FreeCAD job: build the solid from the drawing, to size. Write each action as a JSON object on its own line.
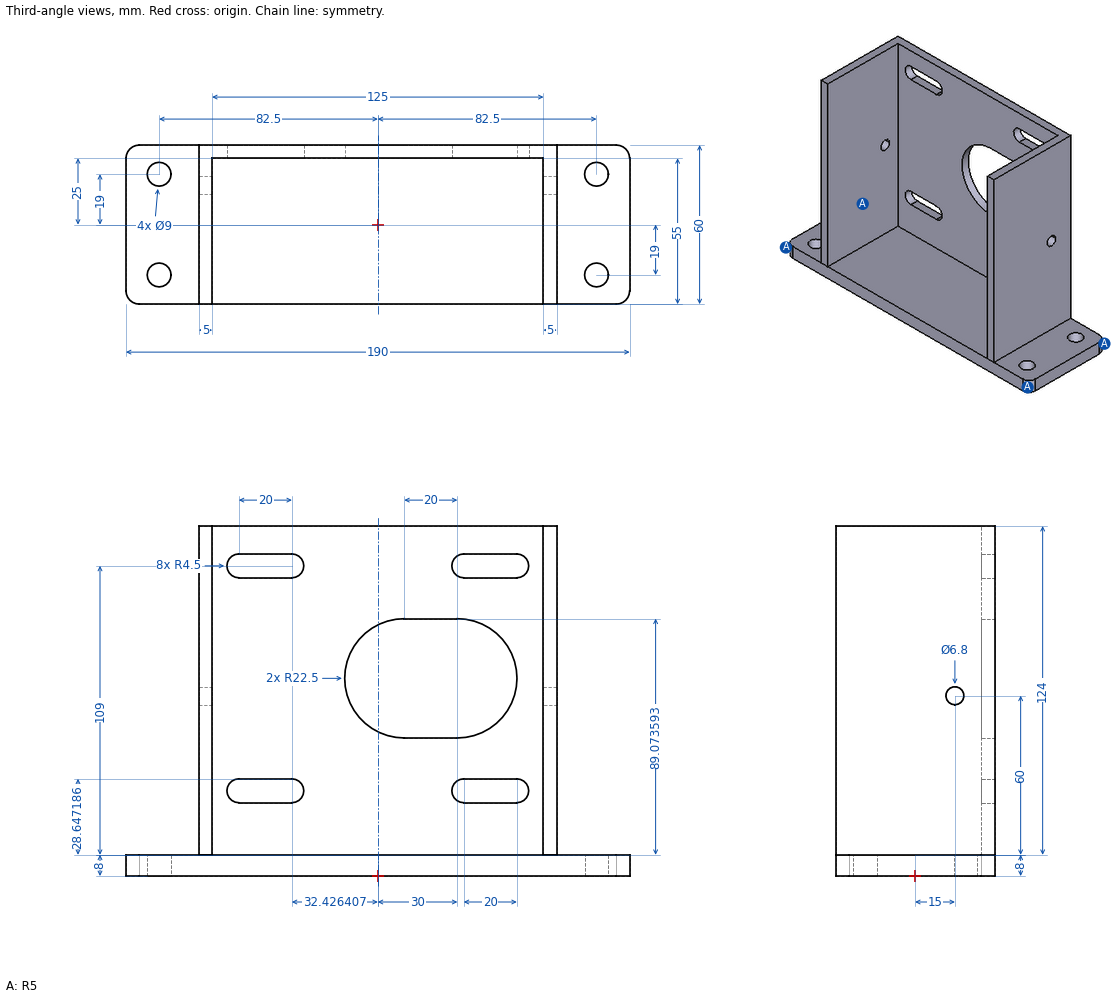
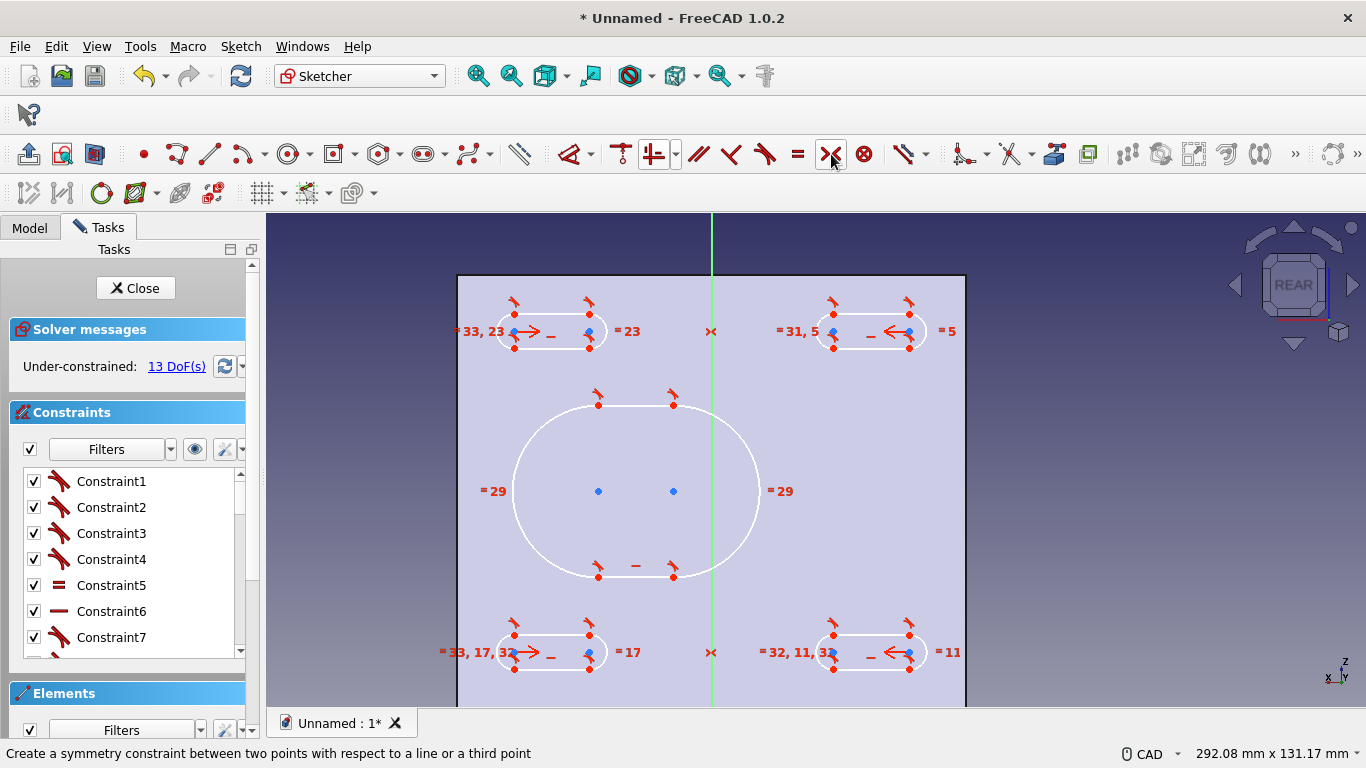
{"action": "left_click", "coordinate": [568, 154]}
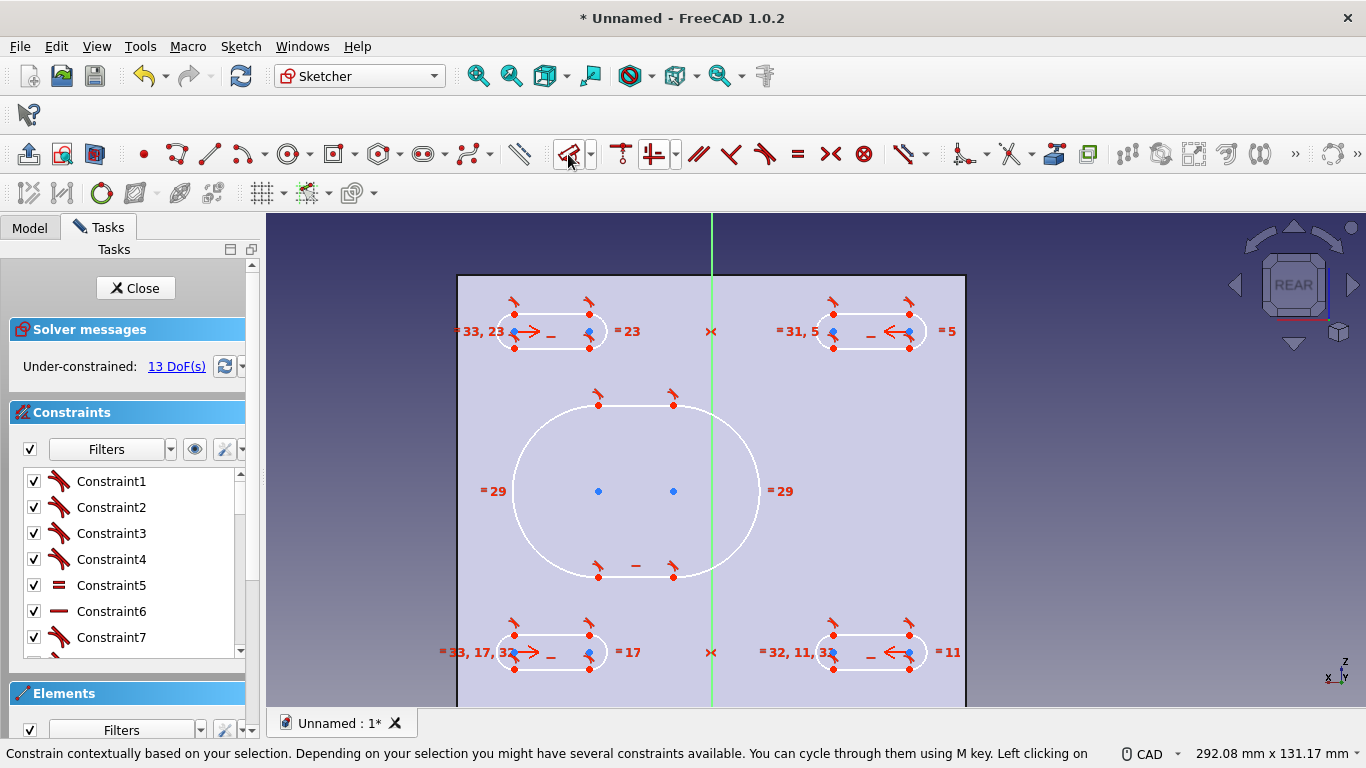
{"action": "scroll", "coordinate": [820, 321], "scroll_direction": "up", "scroll_amount": 5}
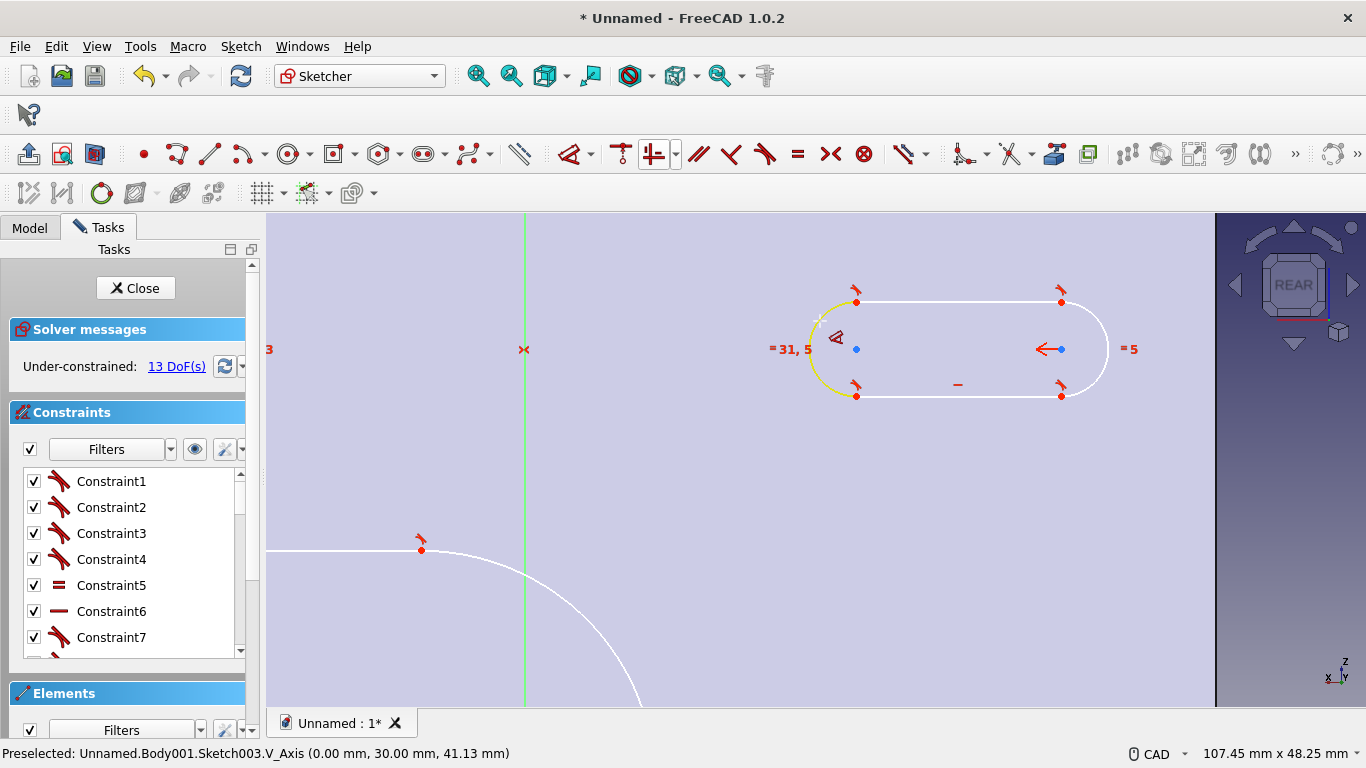
{"action": "left_click", "coordinate": [818, 322]}
{"action": "left_click", "coordinate": [792, 303]}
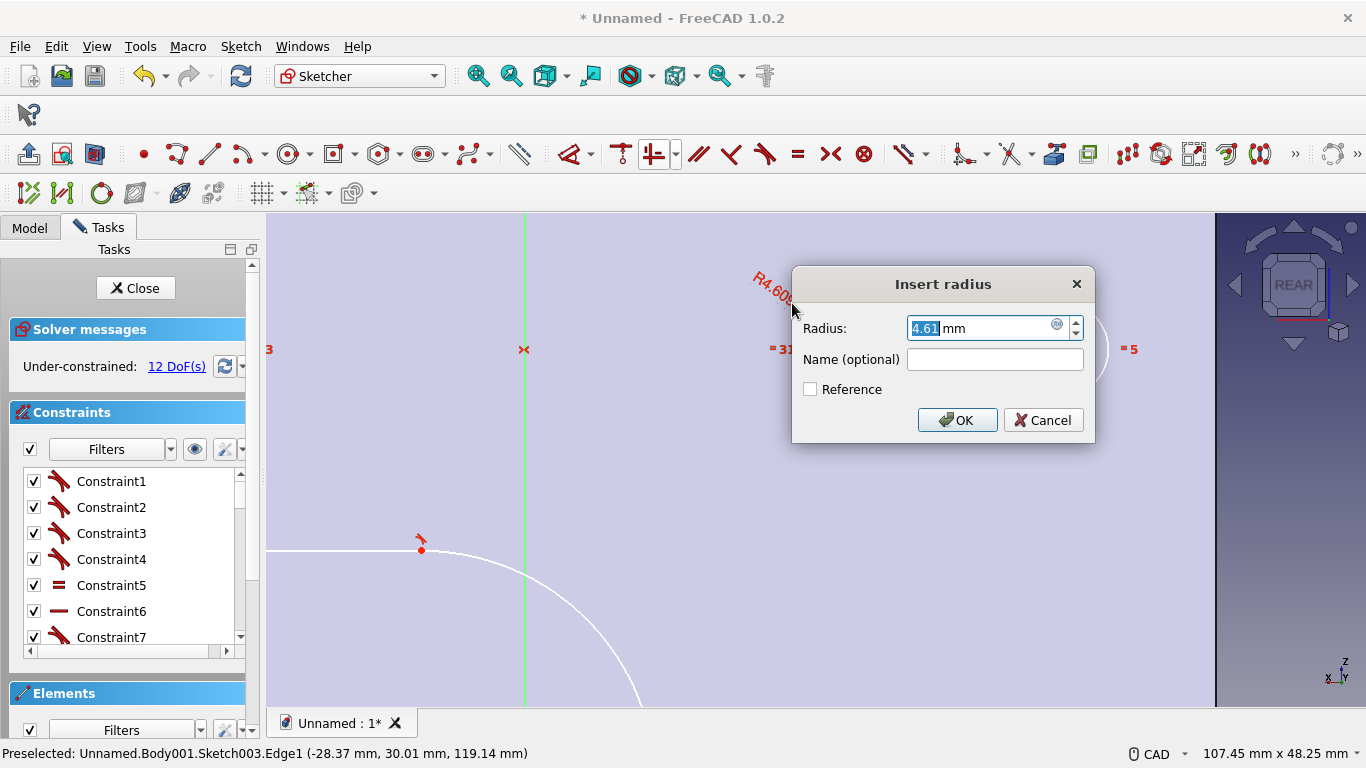
{"action": "type", "text": "4.5"}
{"action": "key", "text": "Return"}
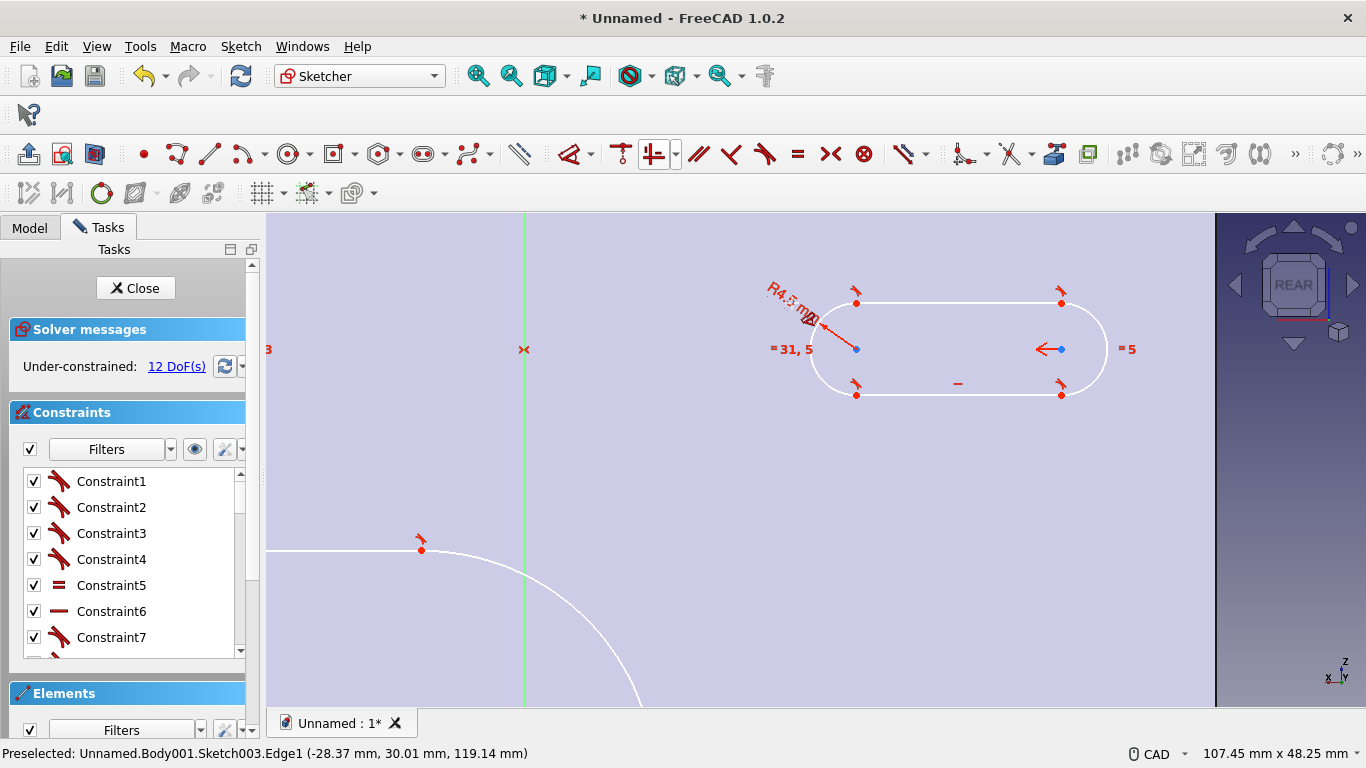
{"action": "scroll", "coordinate": [820, 321], "scroll_direction": "down", "scroll_amount": 7}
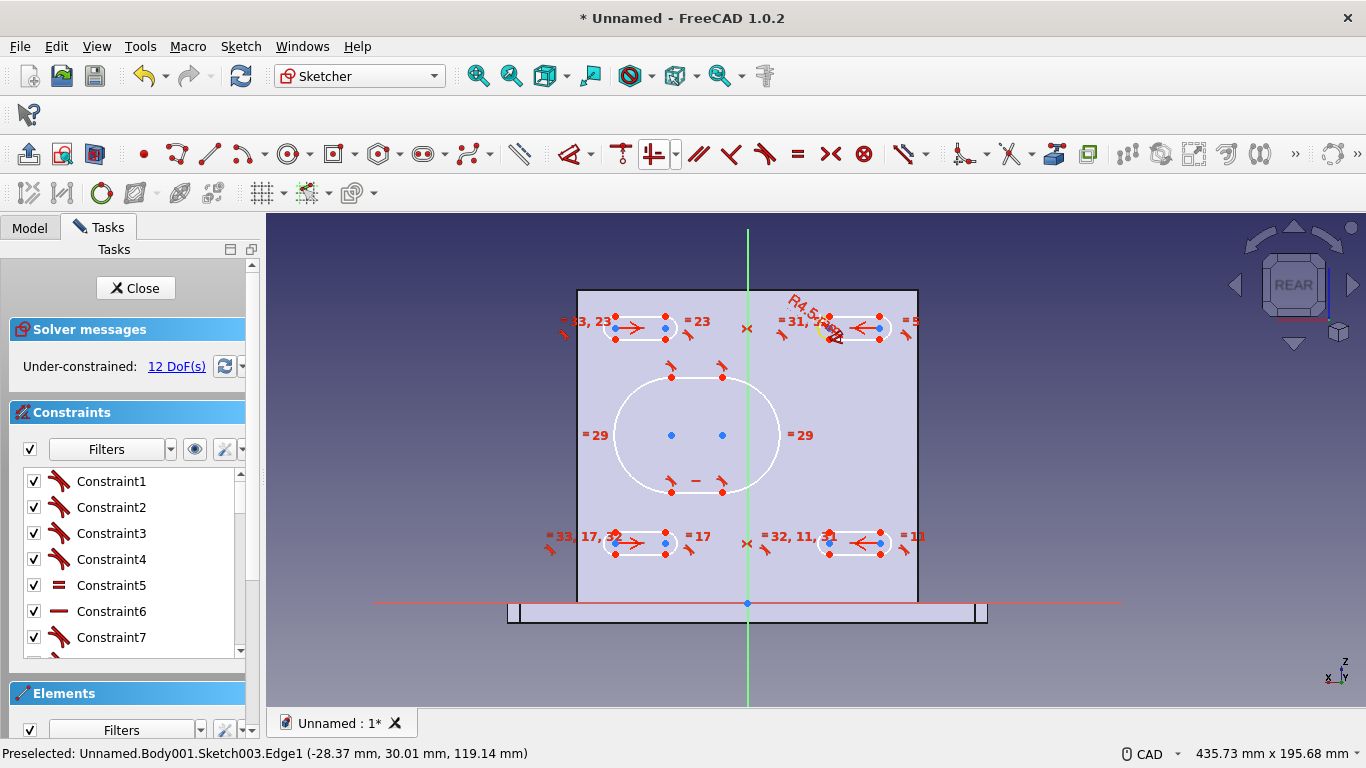
{"action": "left_click", "coordinate": [625, 402]}
{"action": "left_click", "coordinate": [599, 383]}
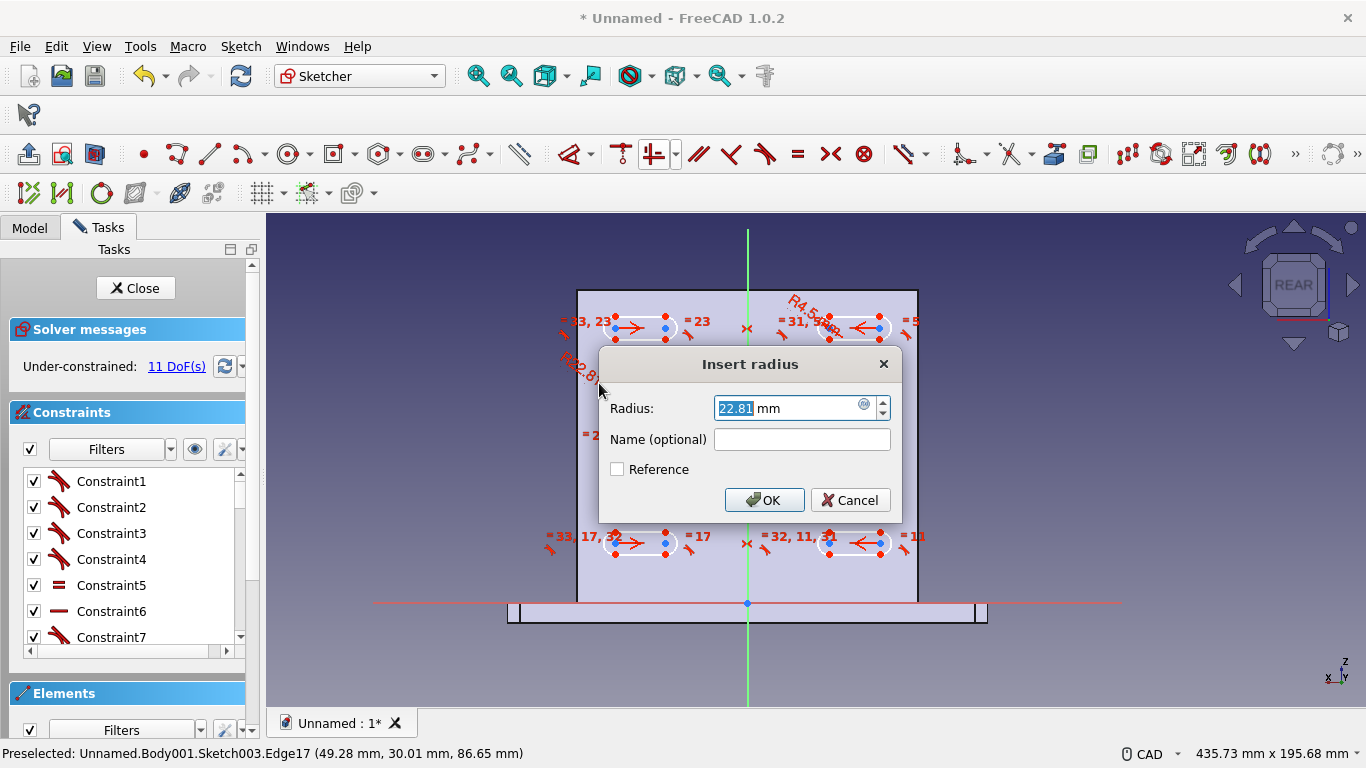
{"action": "type", "text": "22.5"}
{"action": "key", "text": "Return"}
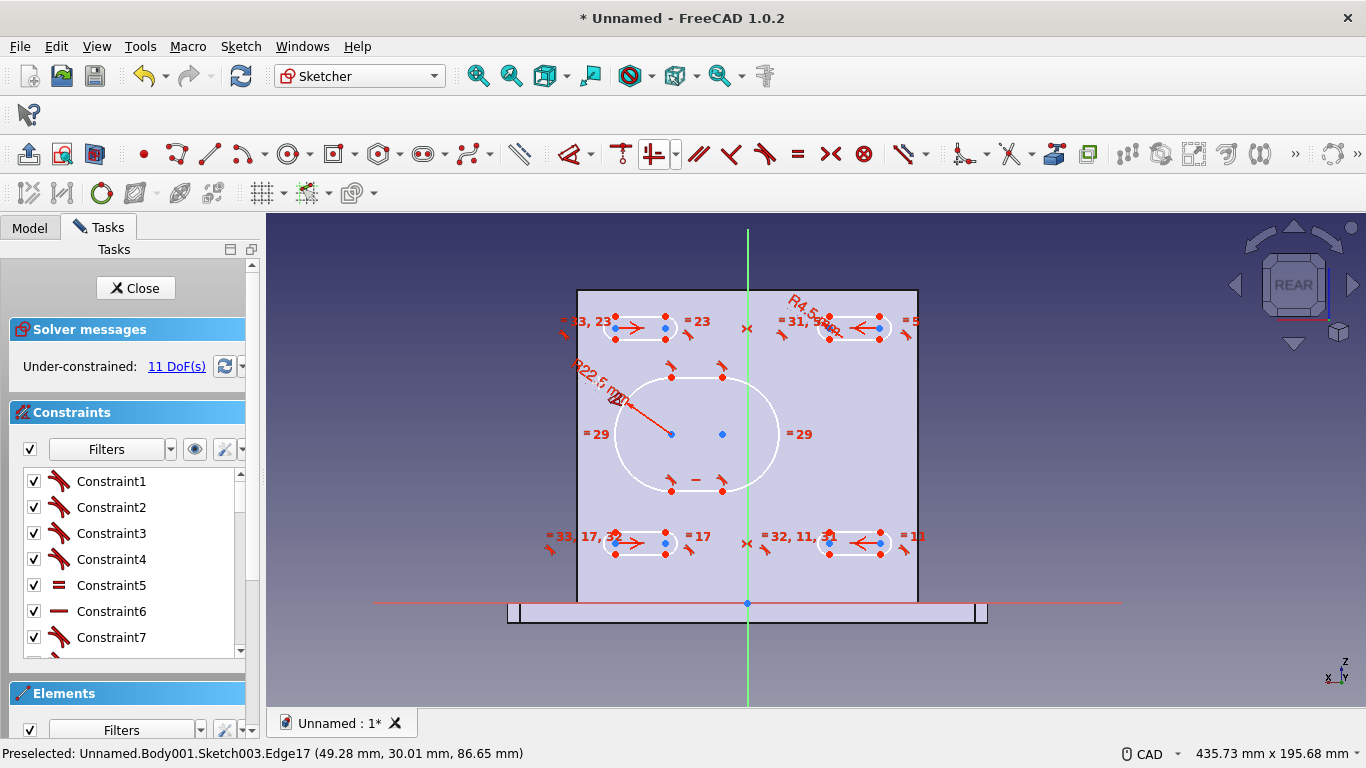
{"action": "left_click", "coordinate": [845, 317]}
{"action": "left_click", "coordinate": [855, 283]}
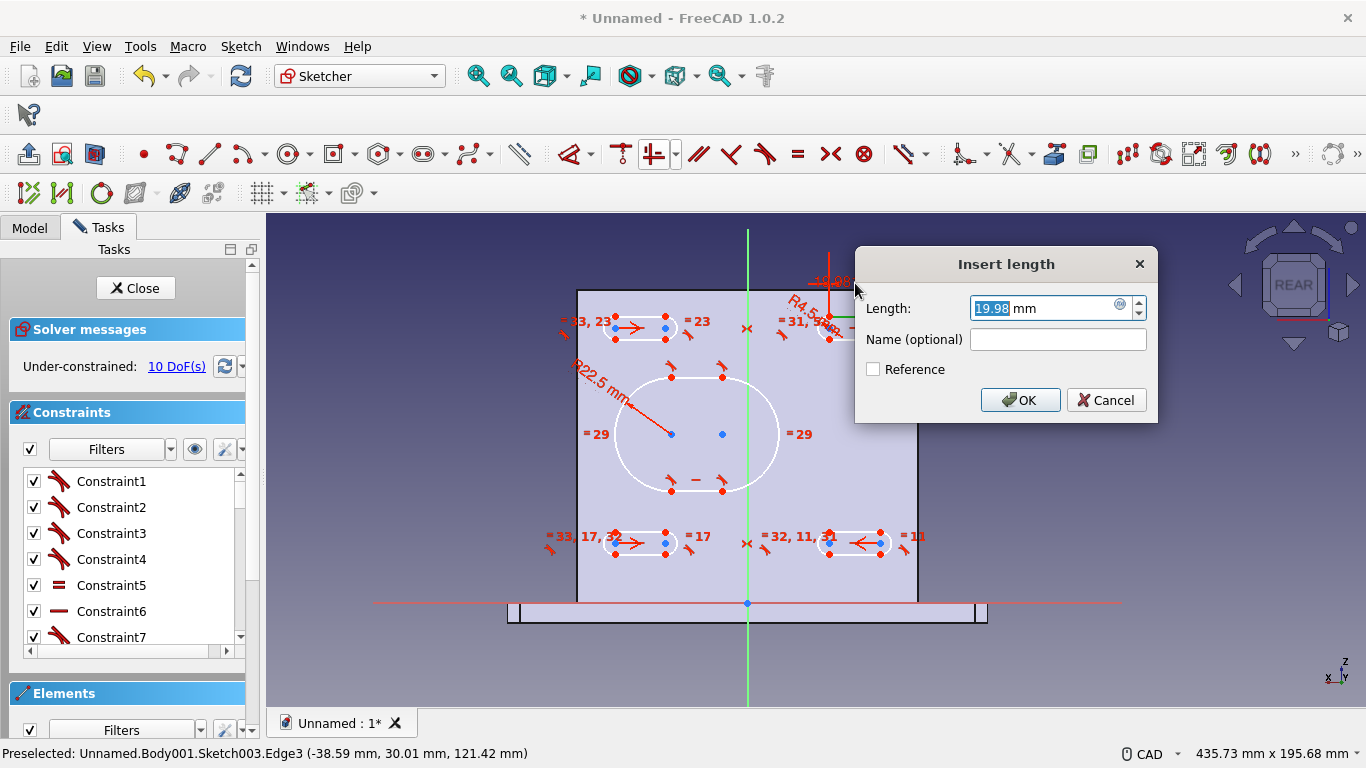
{"action": "type", "text": "20"}
{"action": "key", "text": "Return"}